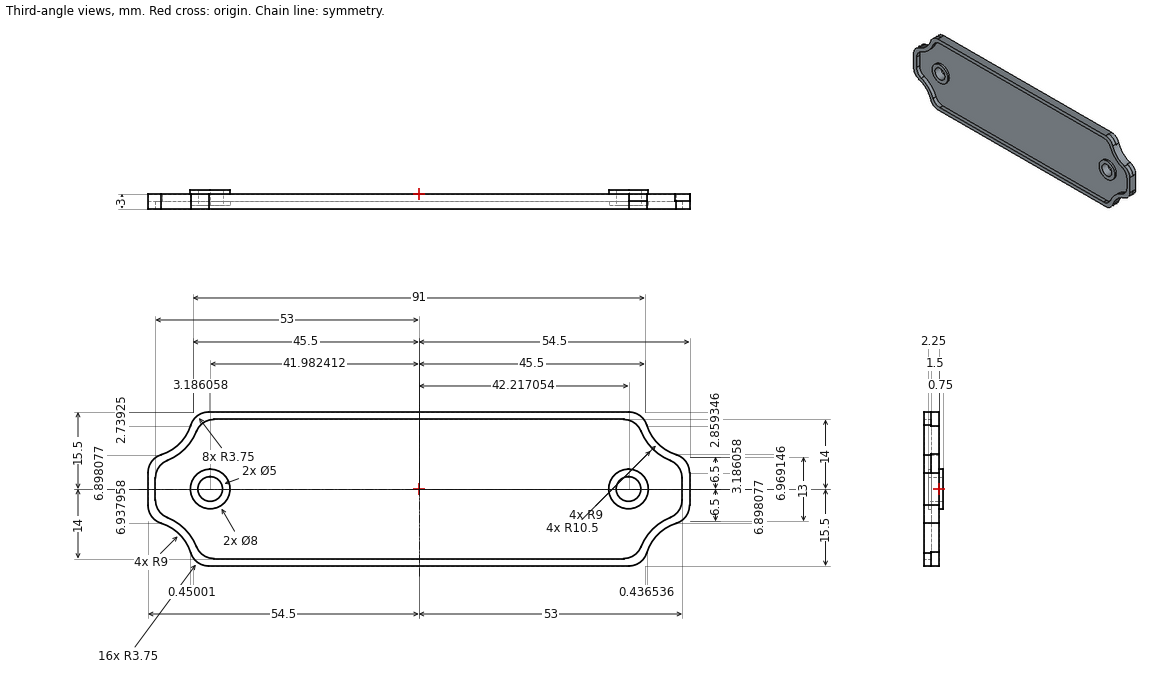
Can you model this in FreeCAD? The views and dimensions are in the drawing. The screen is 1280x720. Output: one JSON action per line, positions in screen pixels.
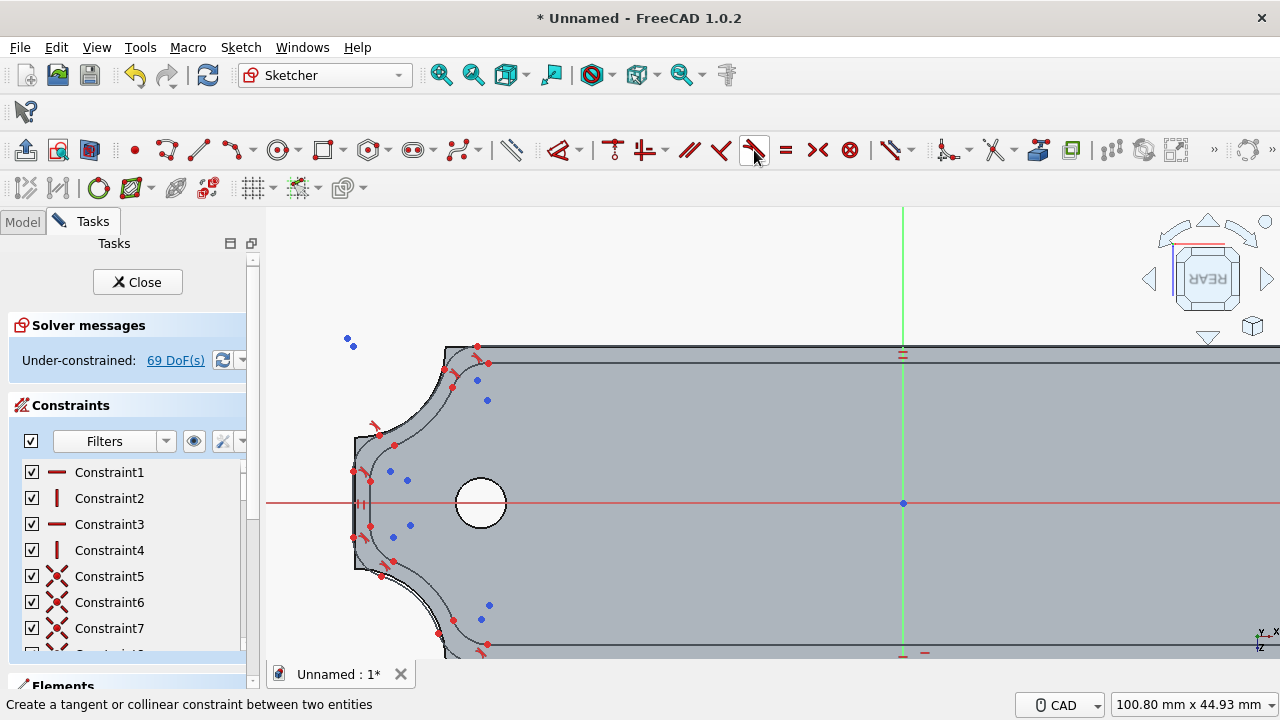
{"action": "left_click", "coordinate": [428, 611]}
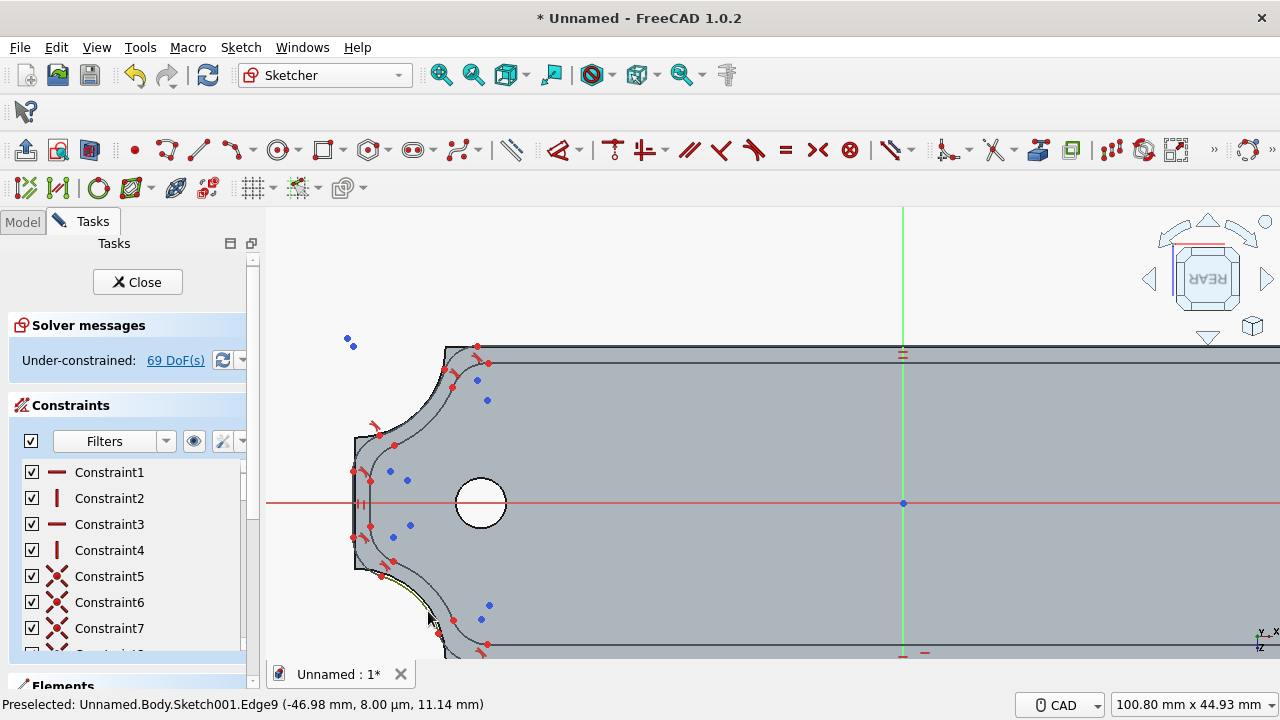
{"action": "scroll", "coordinate": [463, 348], "scroll_direction": "down", "scroll_amount": 3}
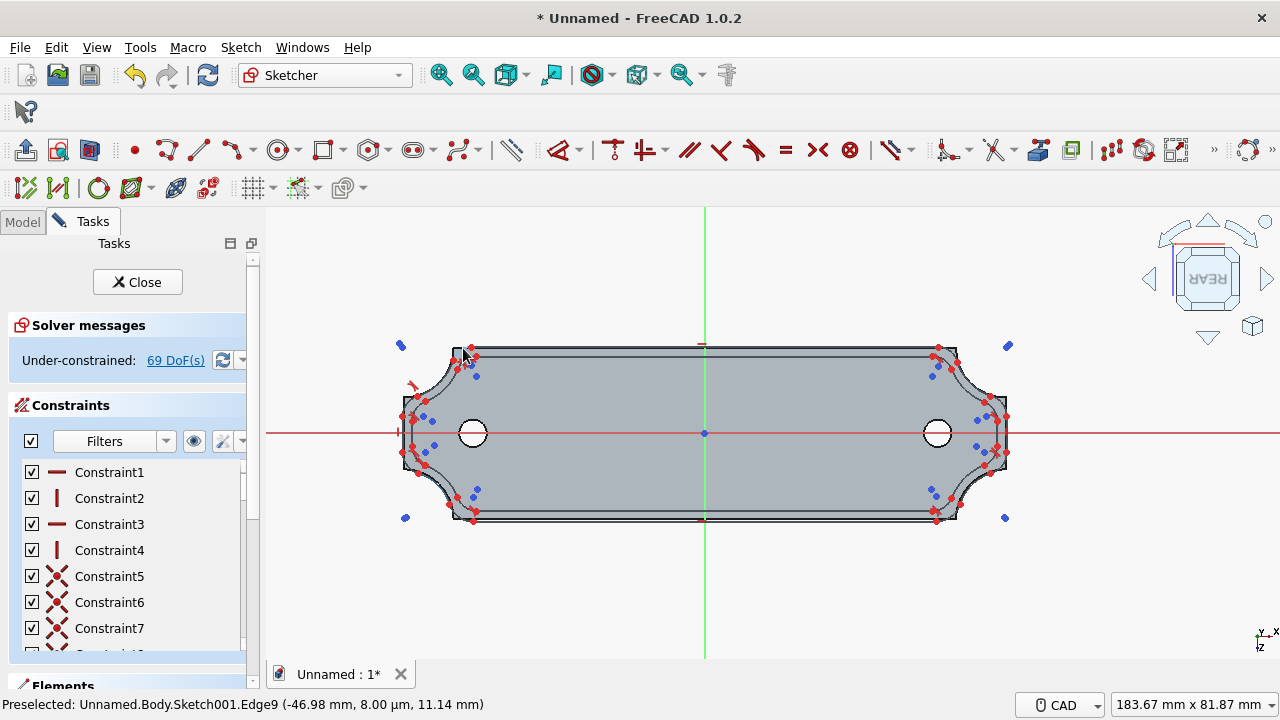
{"action": "scroll", "coordinate": [454, 513], "scroll_direction": "up", "scroll_amount": 3}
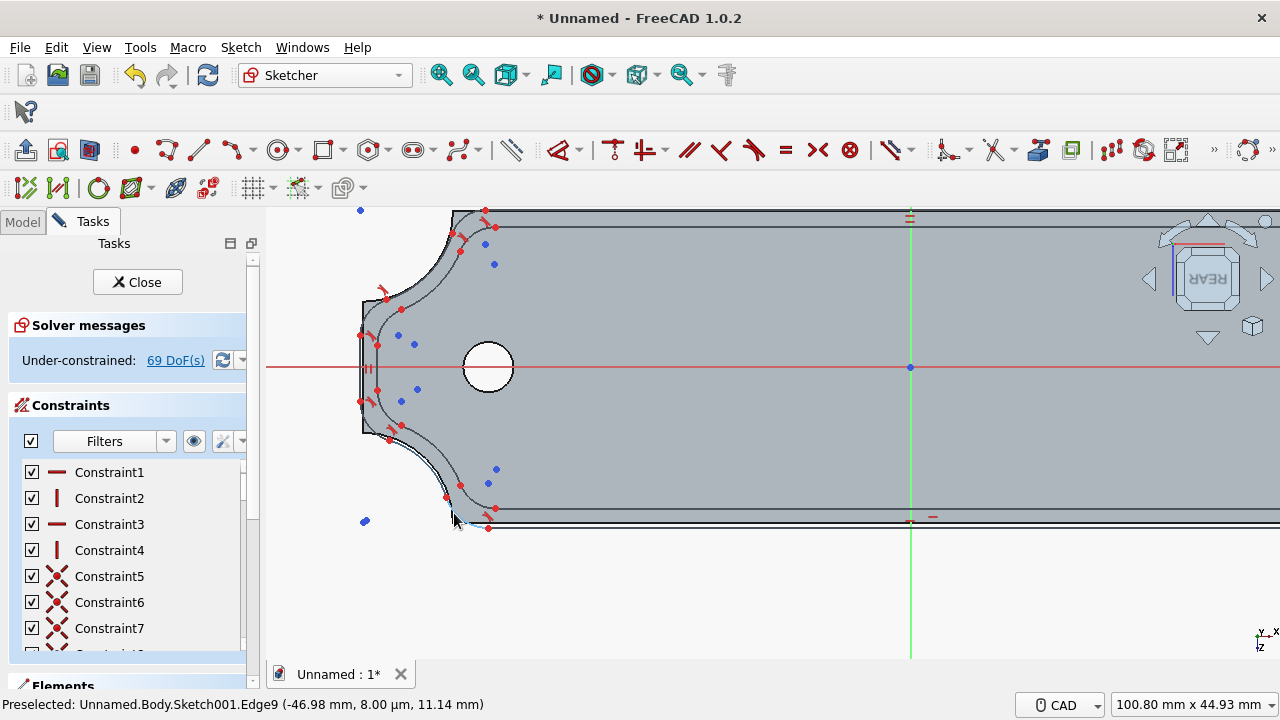
{"action": "left_click", "coordinate": [454, 512]}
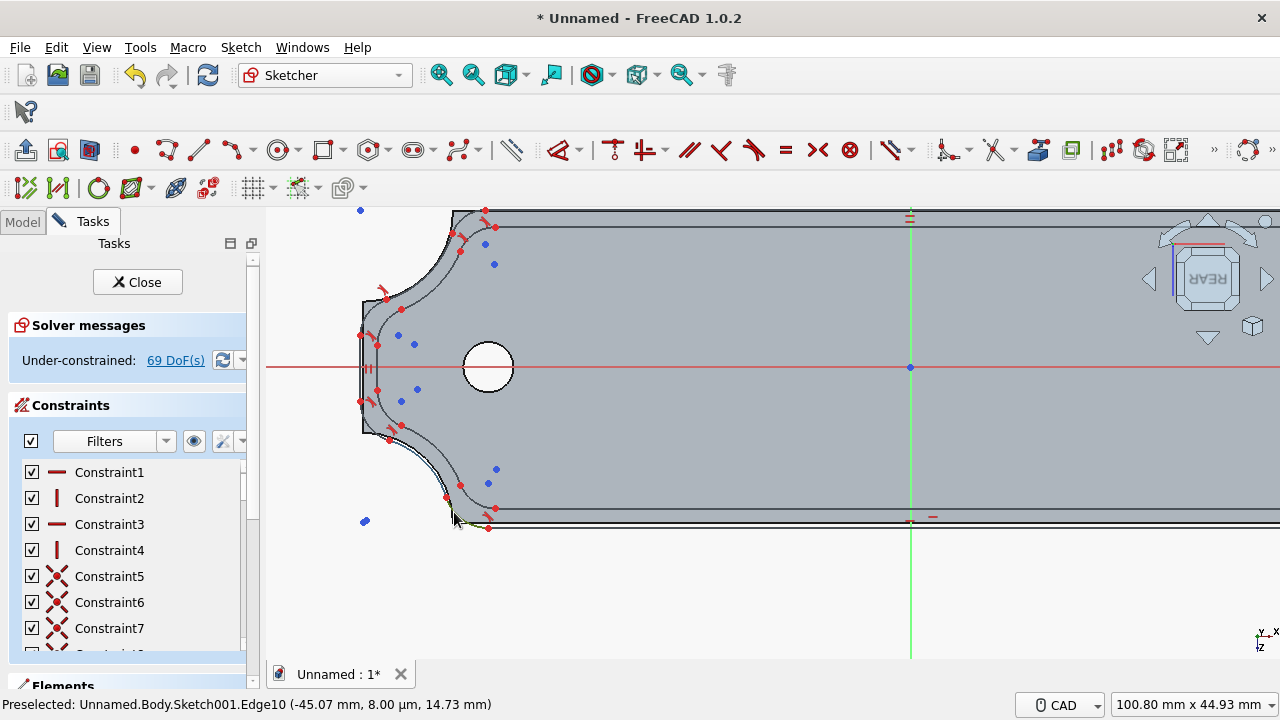
{"action": "left_click", "coordinate": [754, 150]}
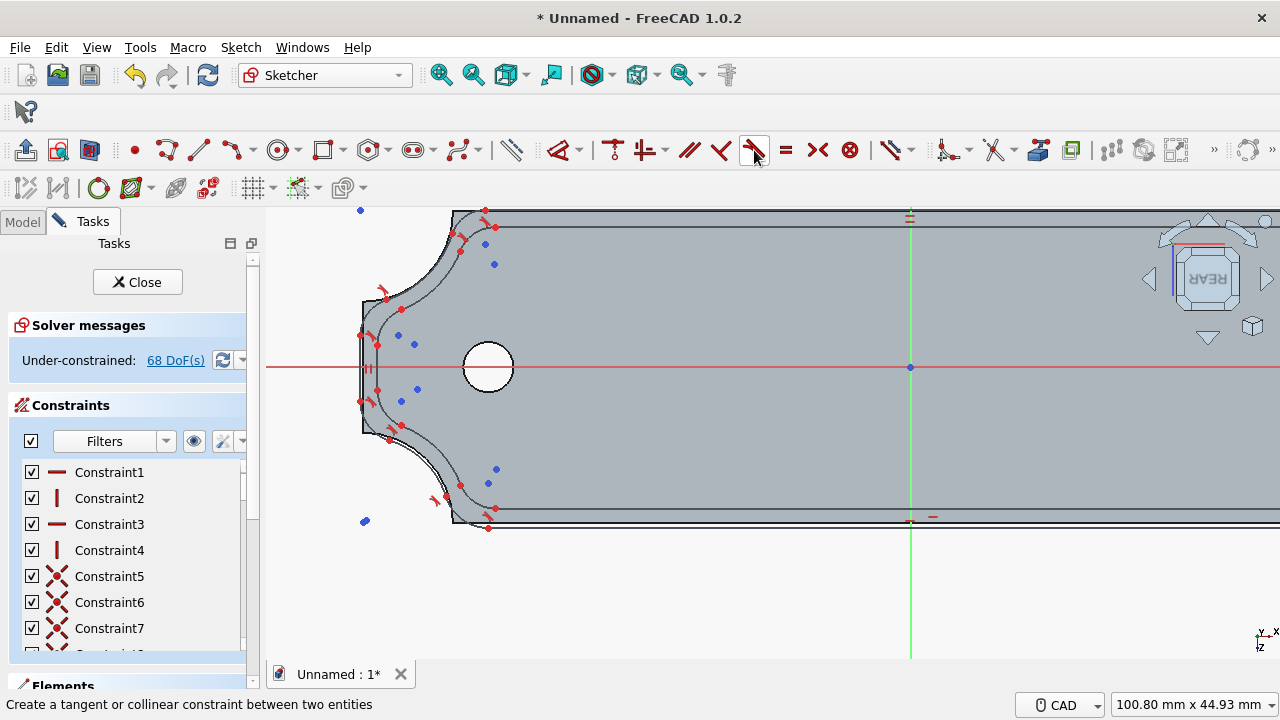
{"action": "scroll", "coordinate": [454, 513], "scroll_direction": "down", "scroll_amount": 3}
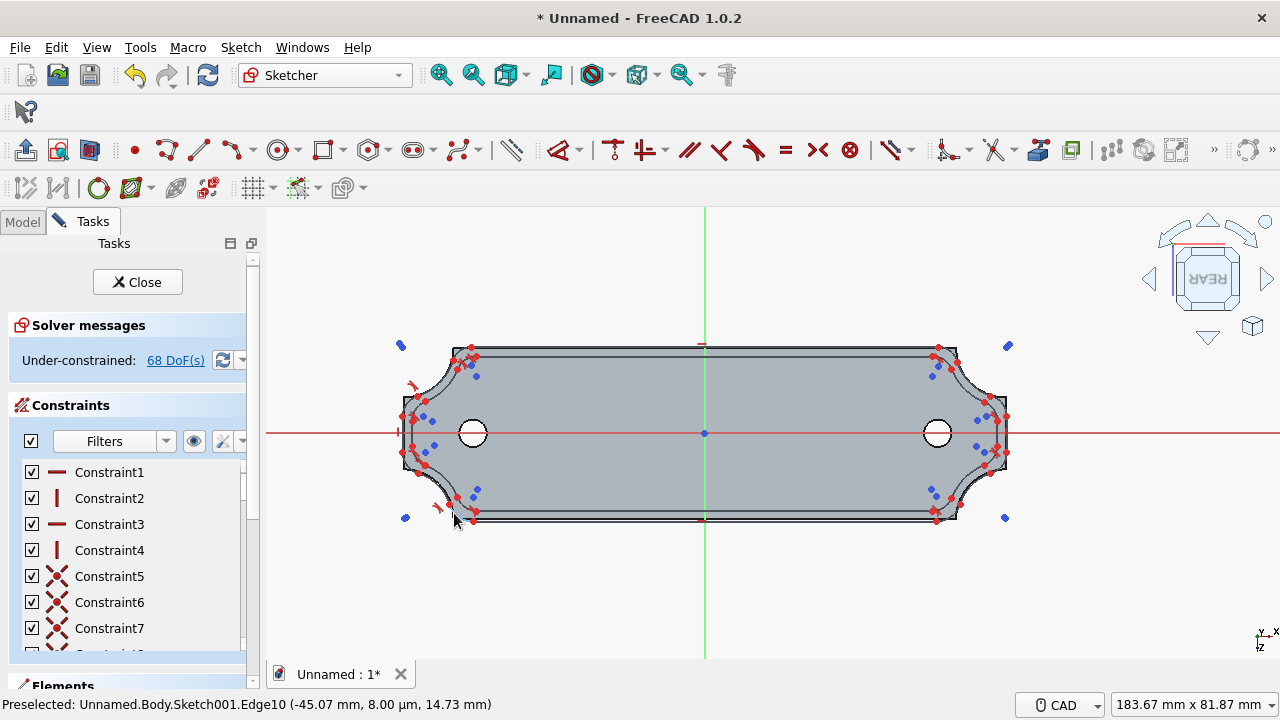
{"action": "scroll", "coordinate": [945, 520], "scroll_direction": "up", "scroll_amount": 3}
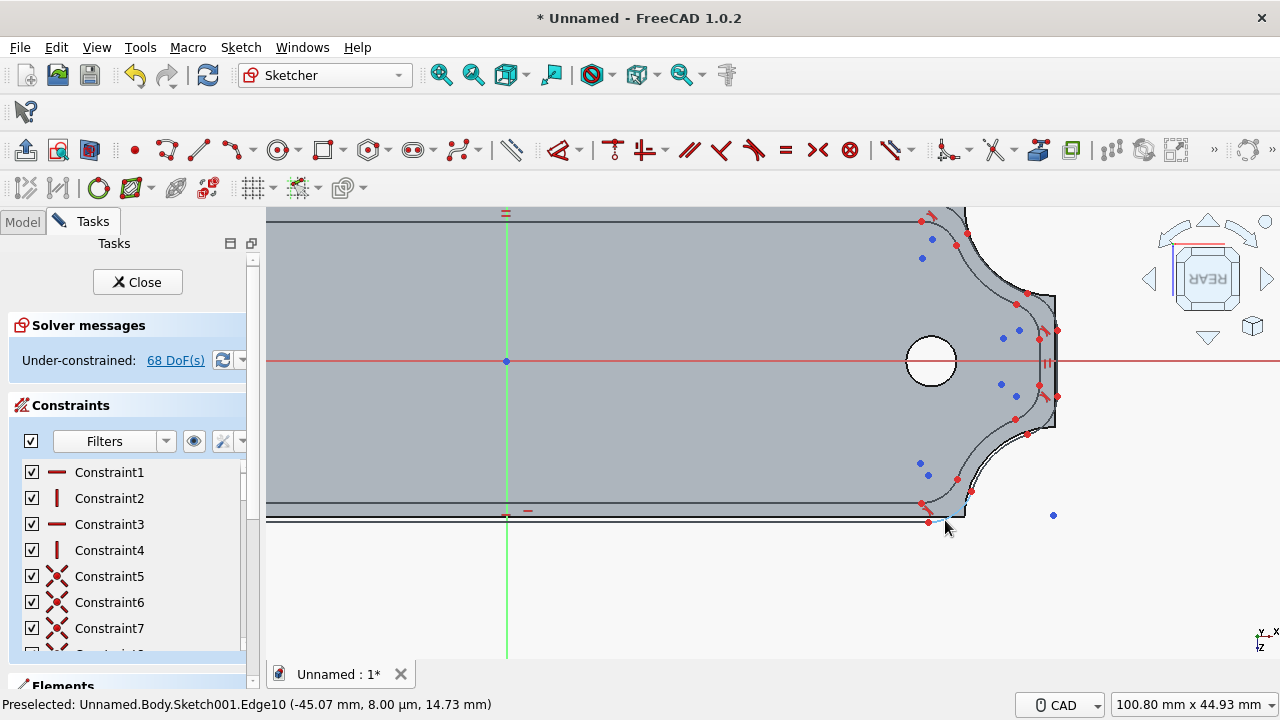
{"action": "left_click", "coordinate": [945, 519]}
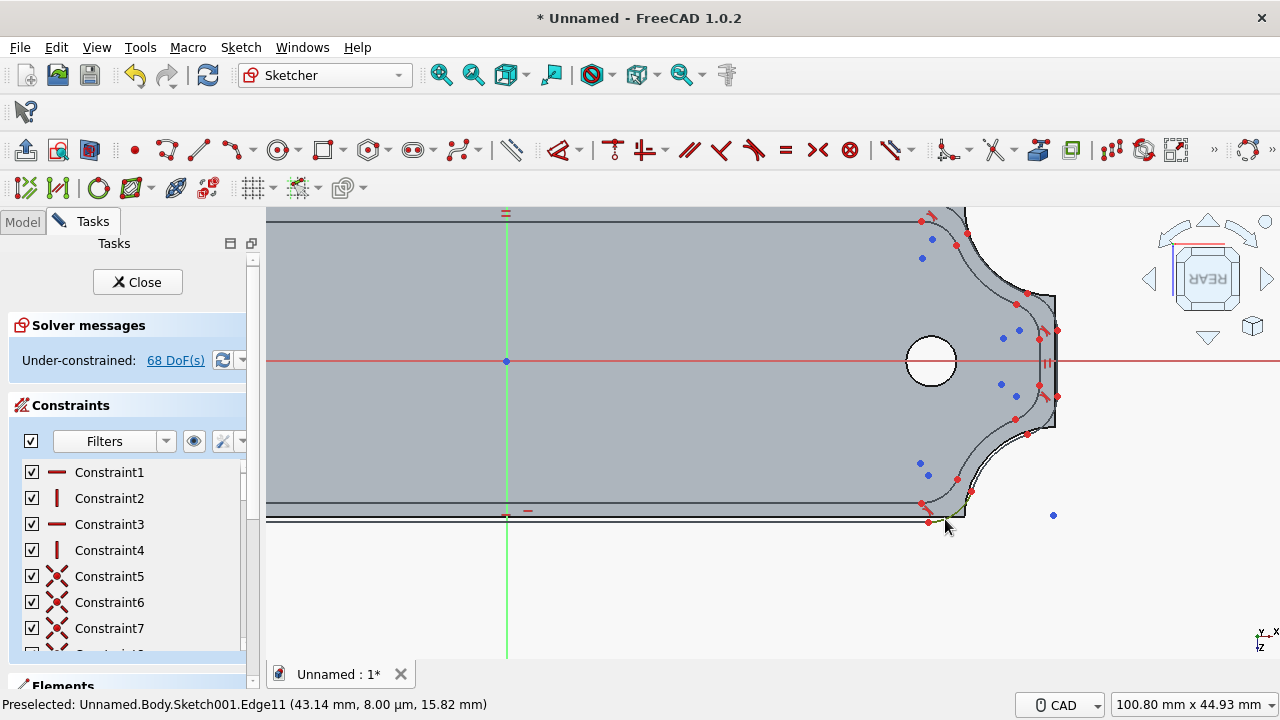
{"action": "left_click", "coordinate": [1005, 446]}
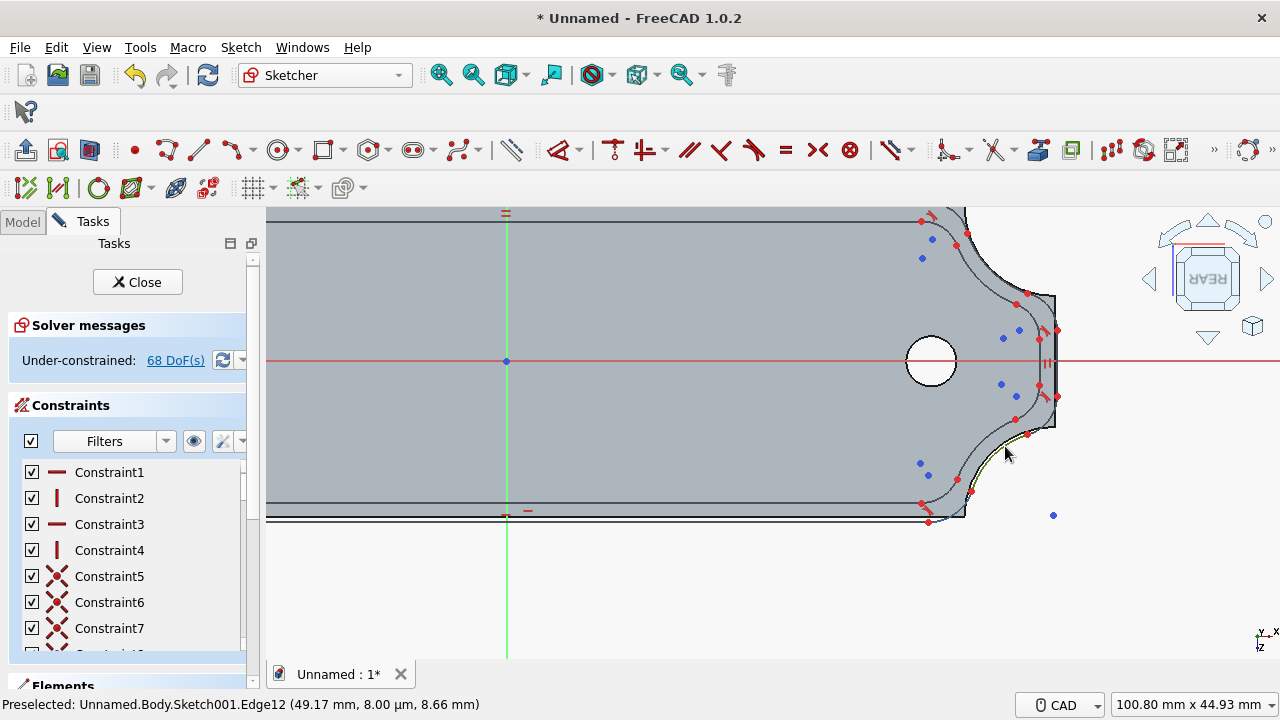
{"action": "left_click", "coordinate": [754, 150]}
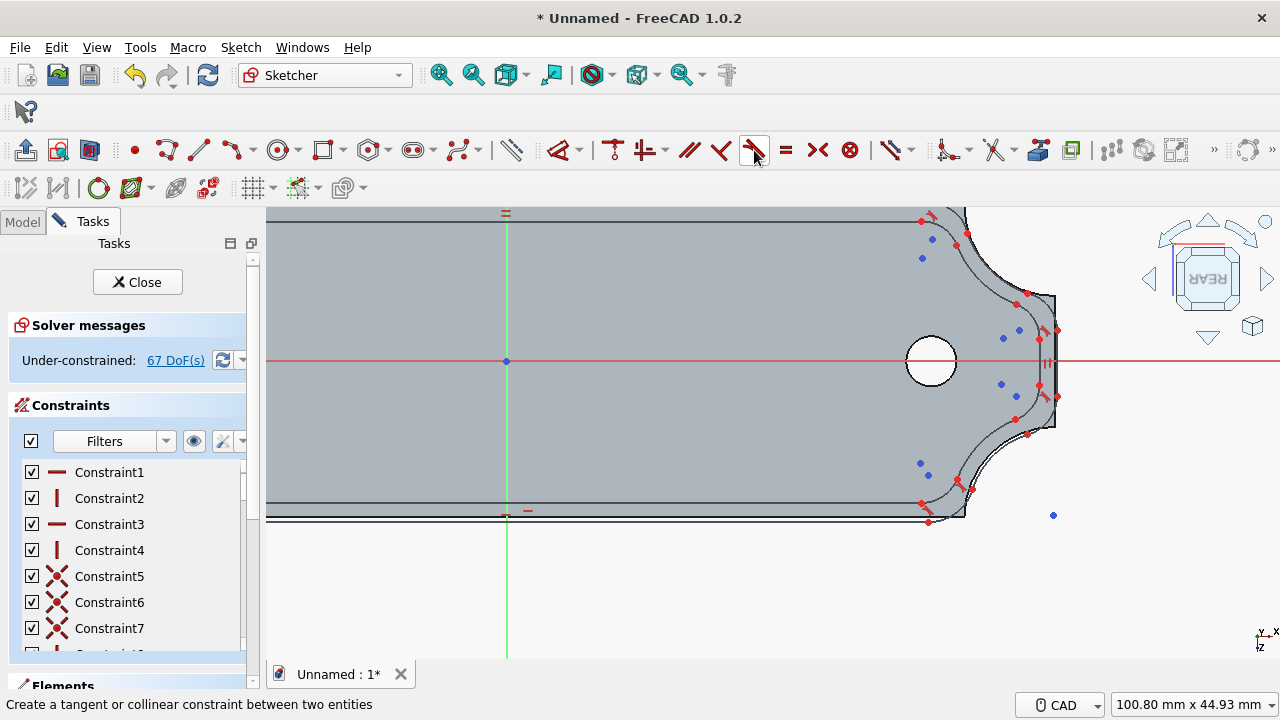
{"action": "left_click", "coordinate": [1006, 445]}